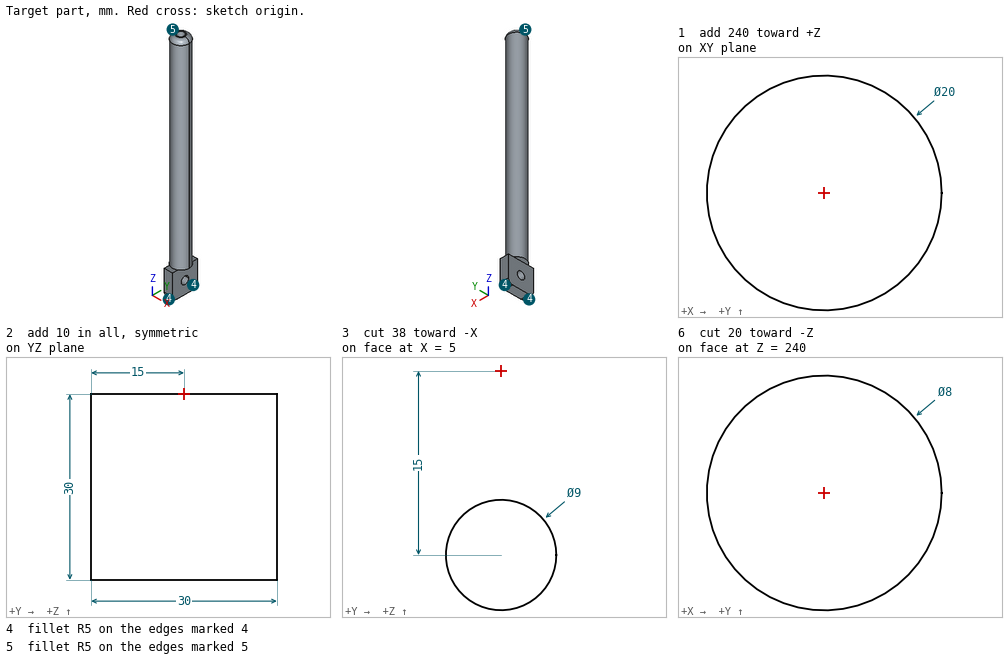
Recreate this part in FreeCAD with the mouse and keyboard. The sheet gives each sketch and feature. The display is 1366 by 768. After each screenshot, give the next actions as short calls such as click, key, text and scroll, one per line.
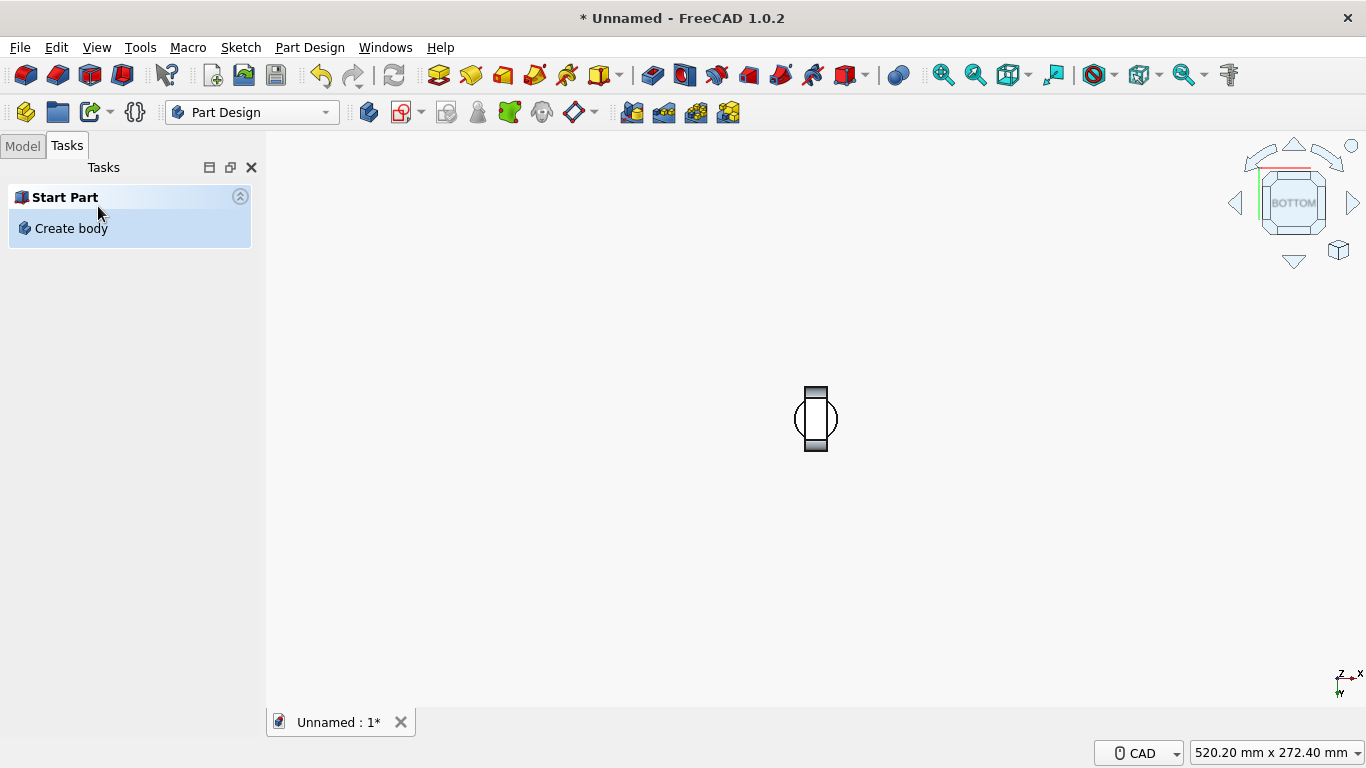
key(v)
key(f)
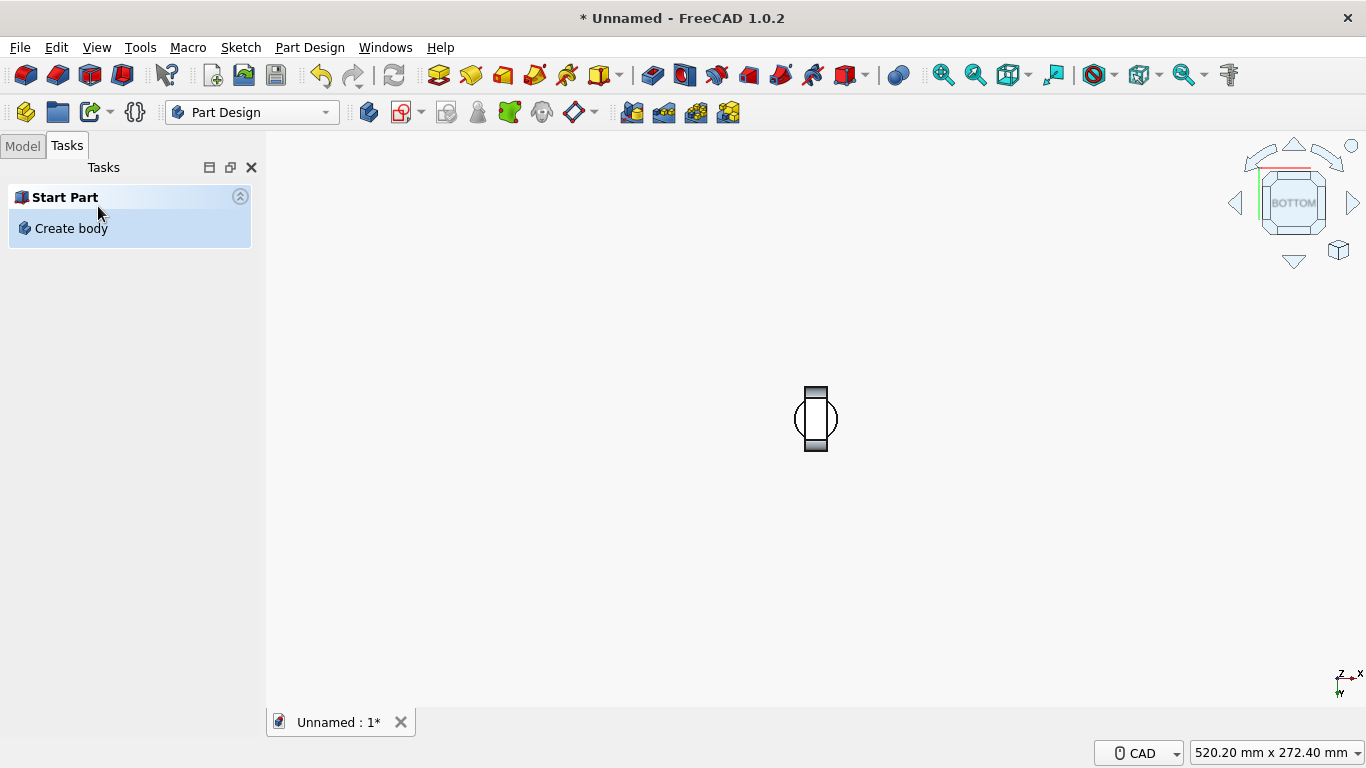
key(0)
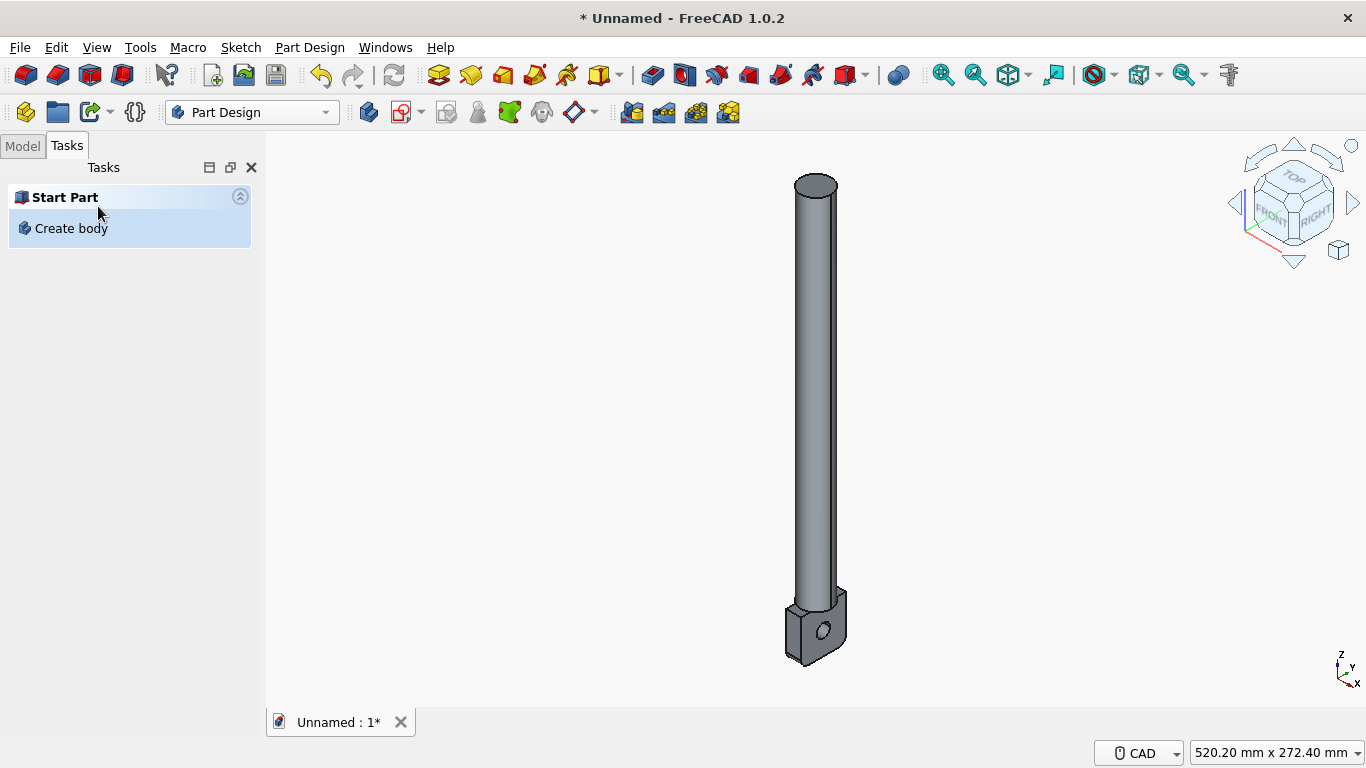
click(795, 183)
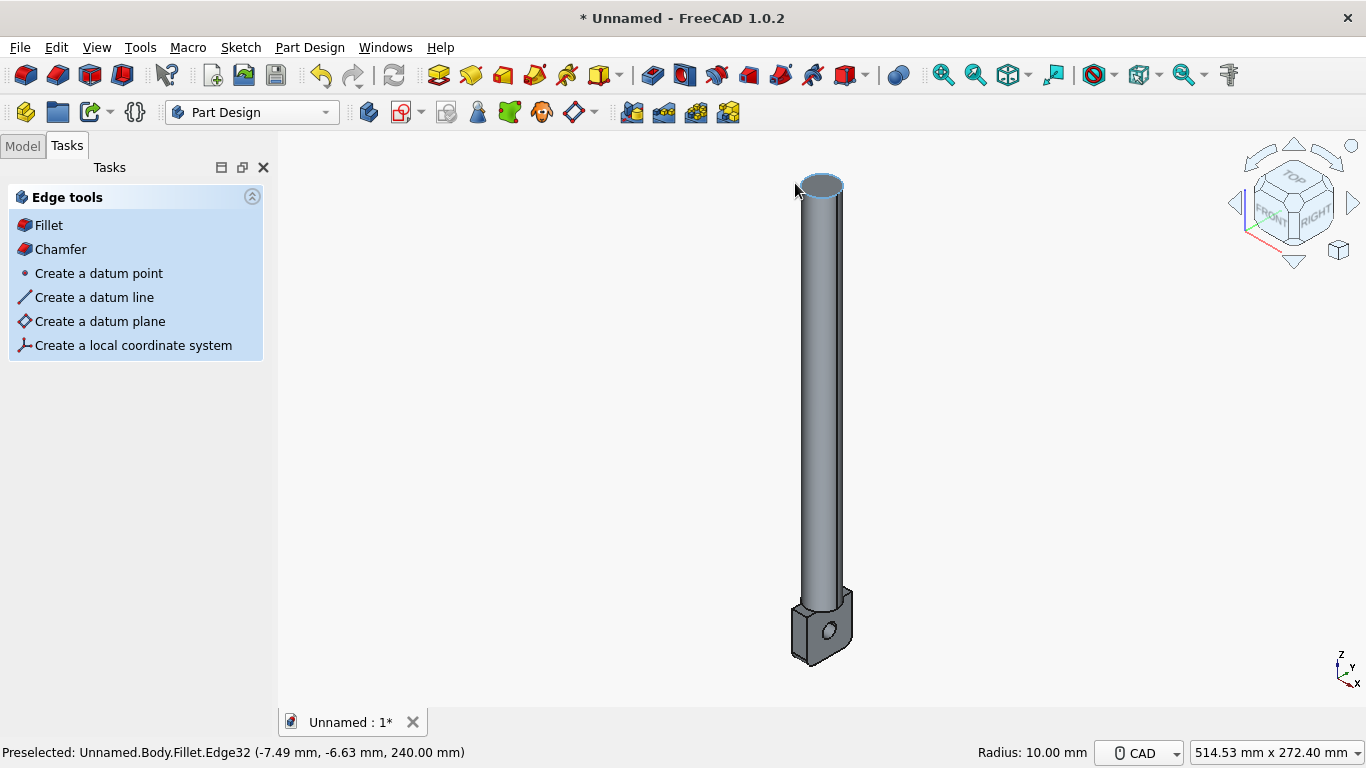
click(26, 76)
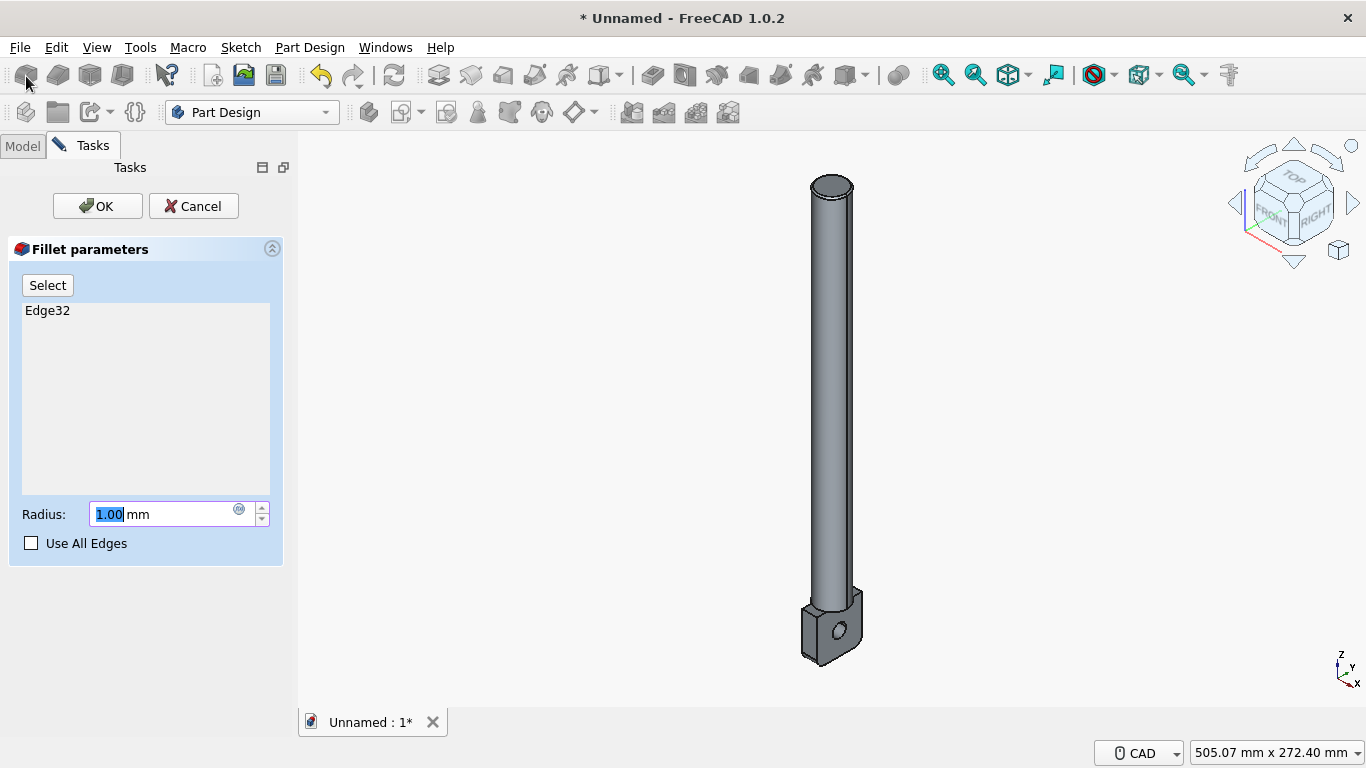
text(5)
key(Tab)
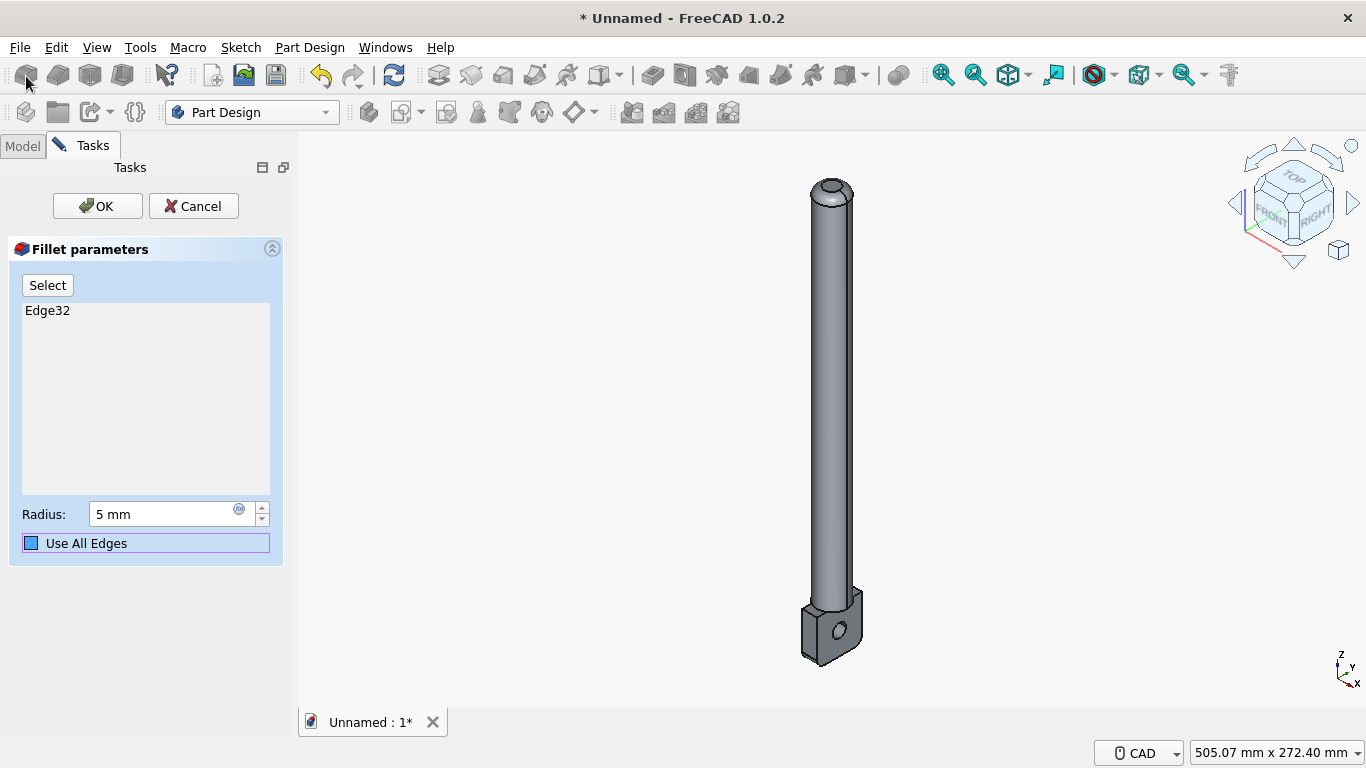
click(98, 206)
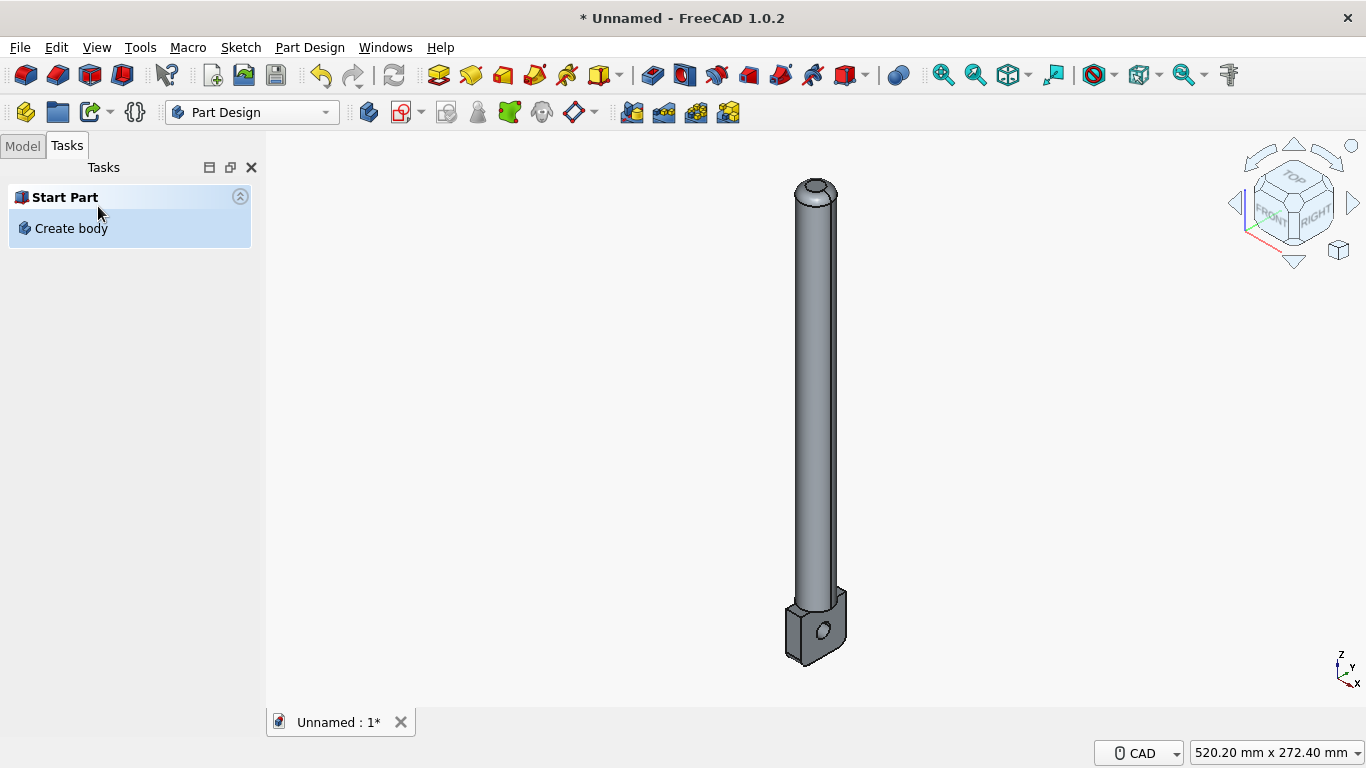
key(2)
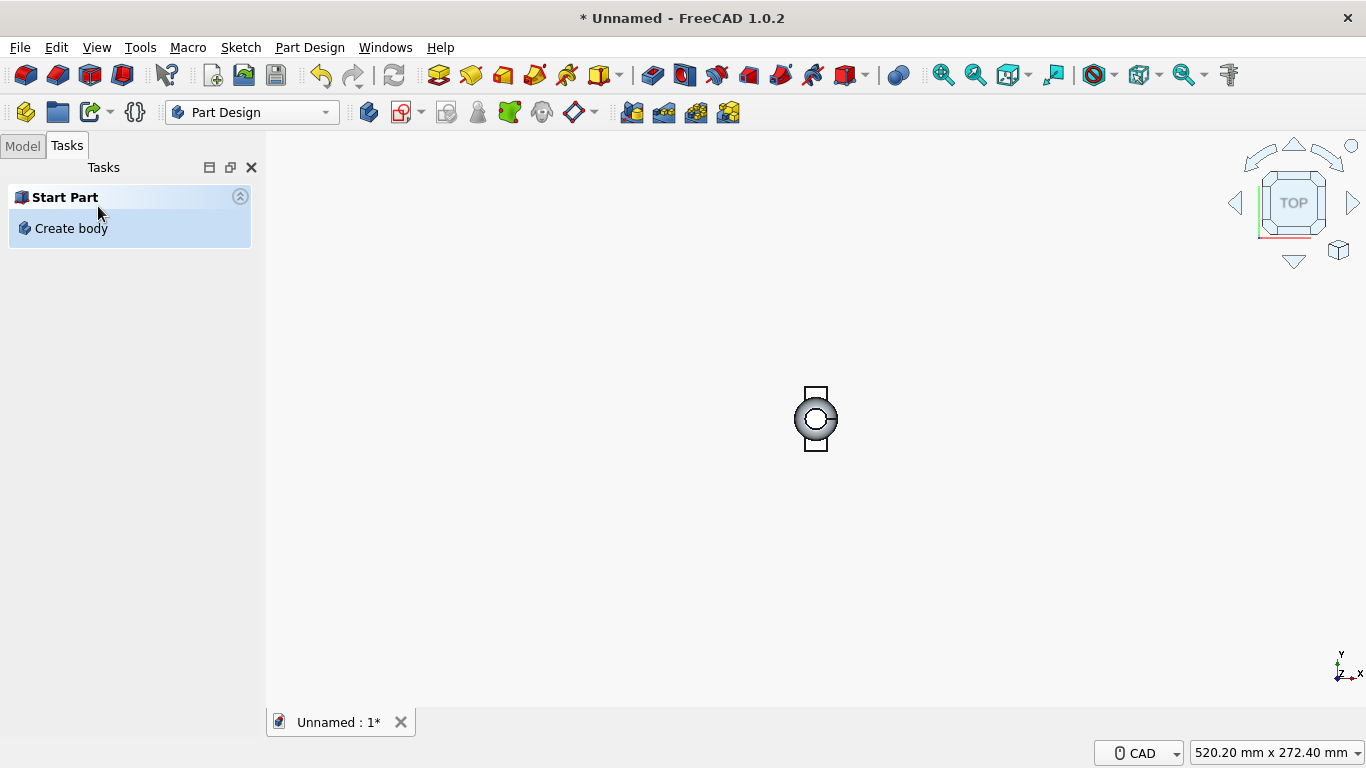
click(944, 76)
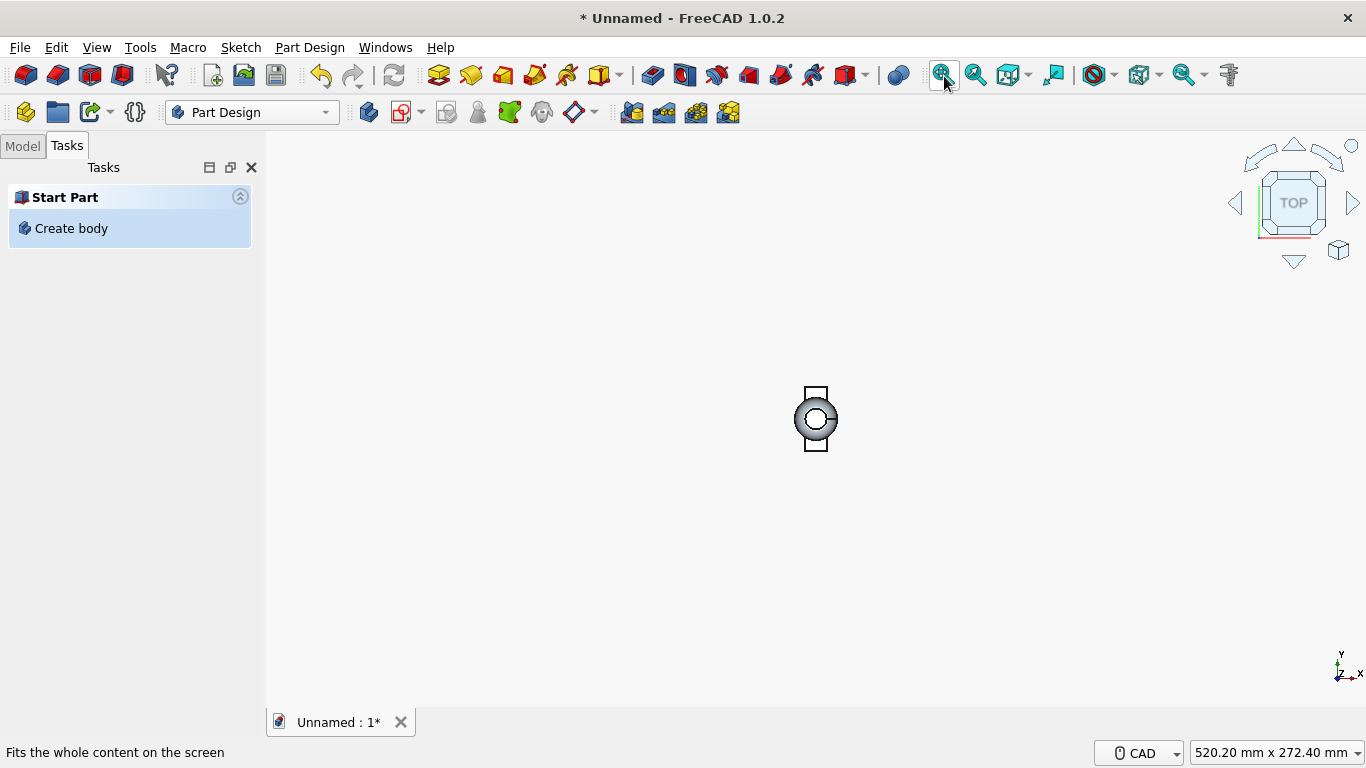
click(816, 418)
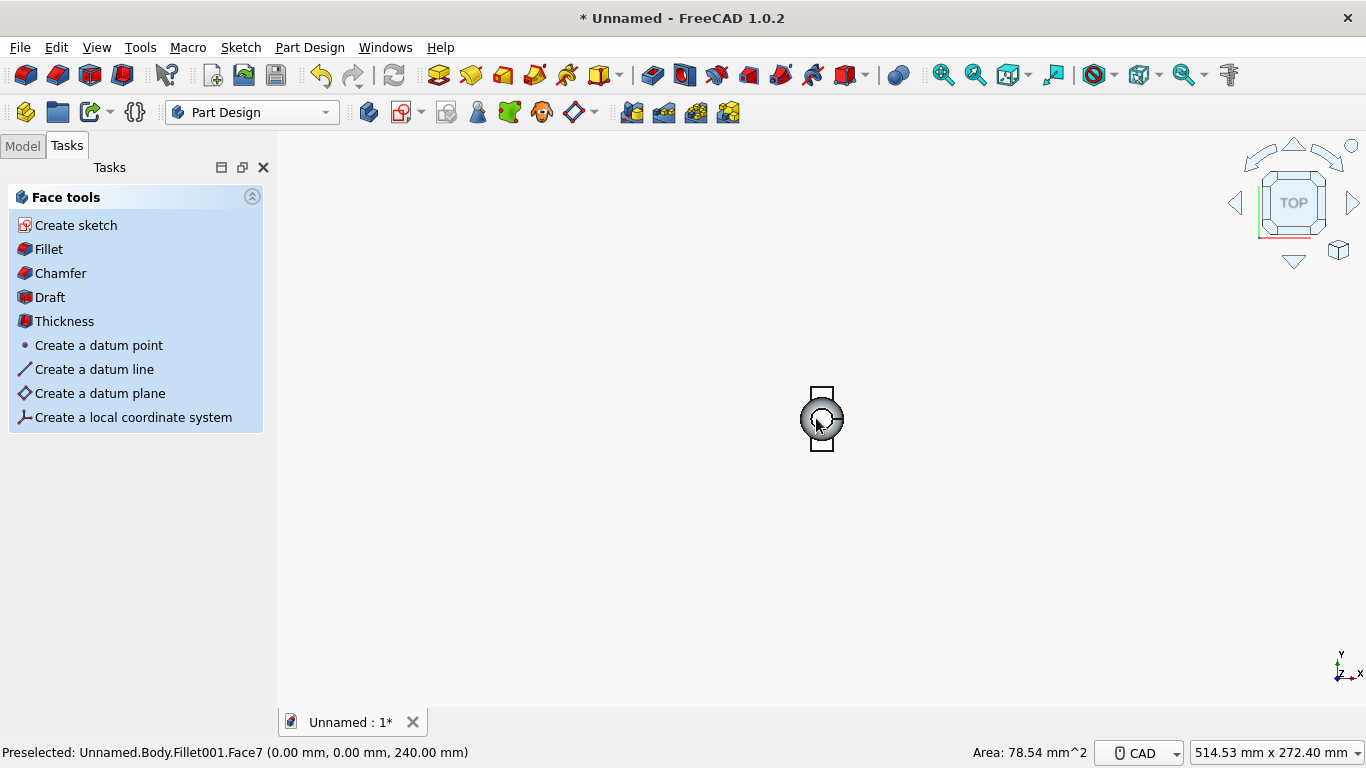
click(402, 112)